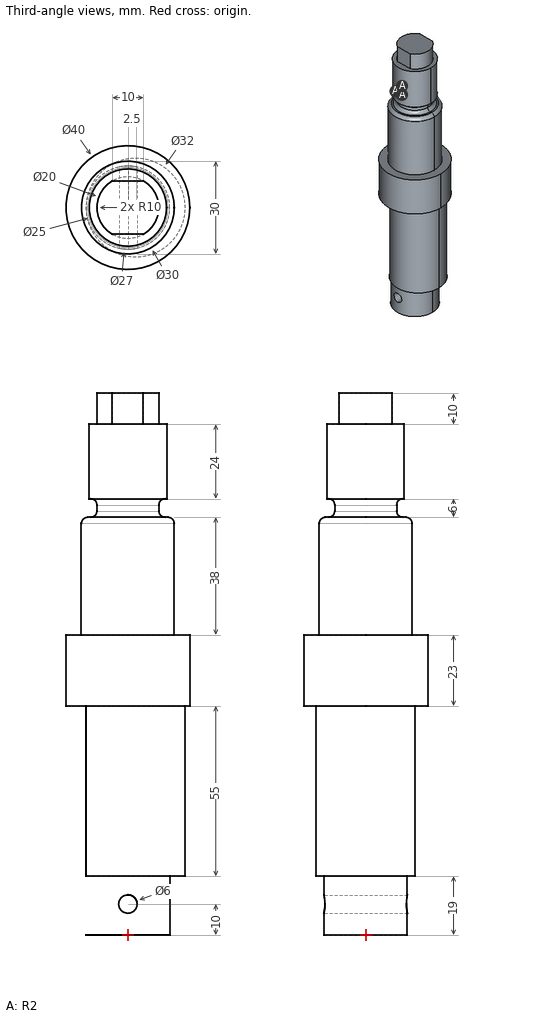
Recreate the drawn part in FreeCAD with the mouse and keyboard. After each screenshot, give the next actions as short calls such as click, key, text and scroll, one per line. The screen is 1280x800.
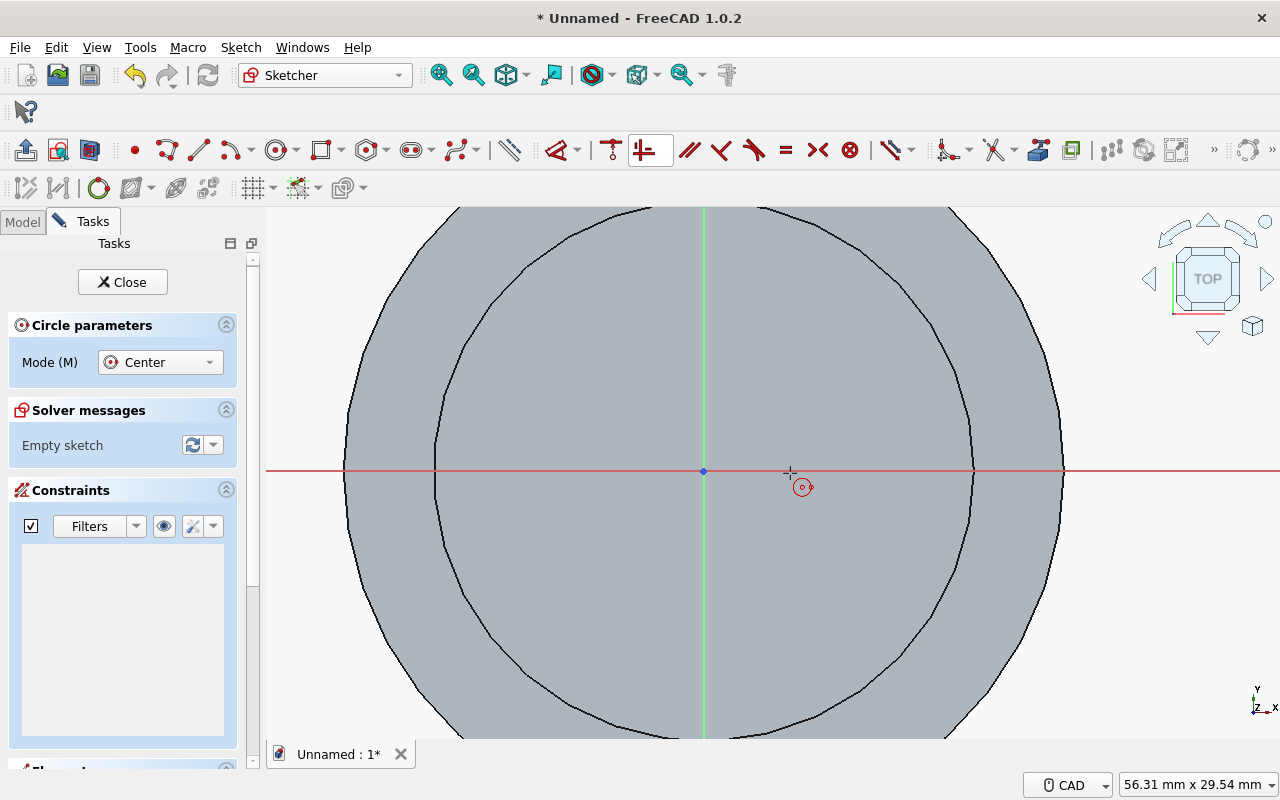
click(704, 471)
click(831, 344)
key(Escape)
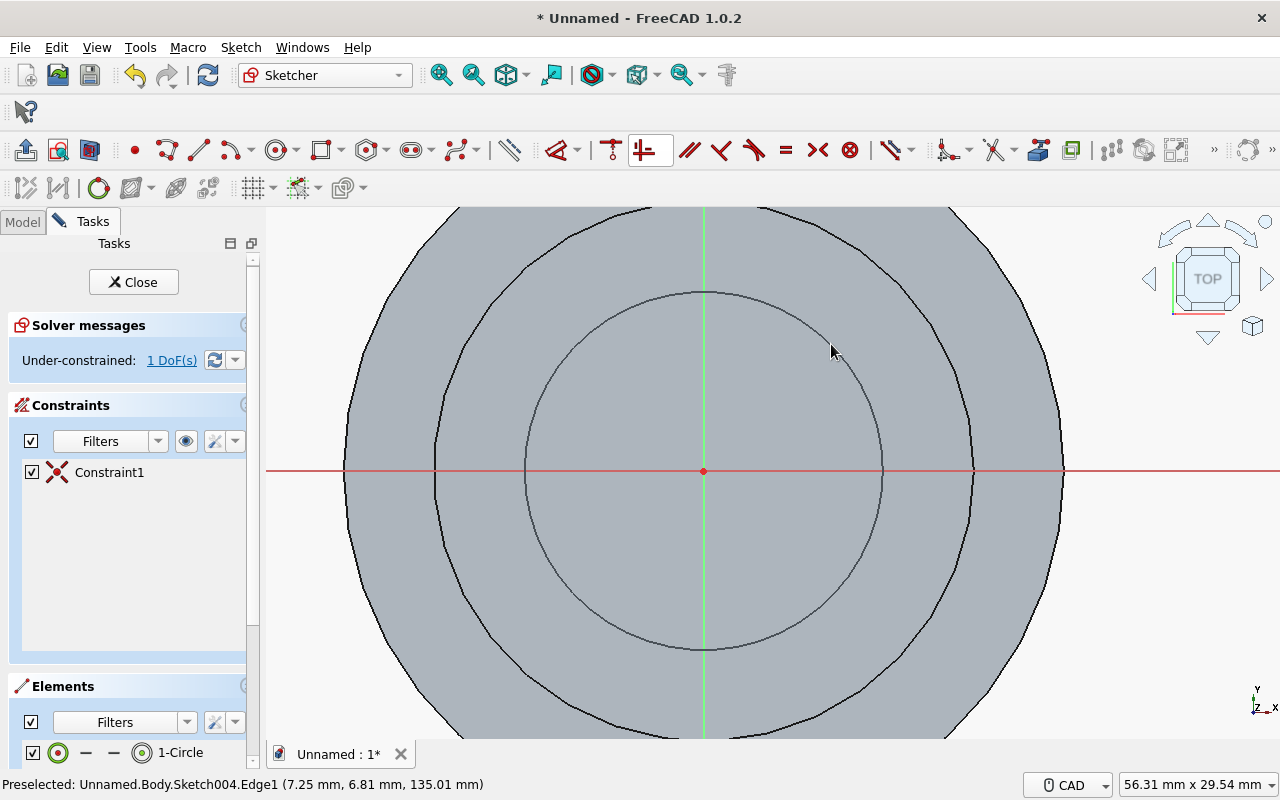
key(d)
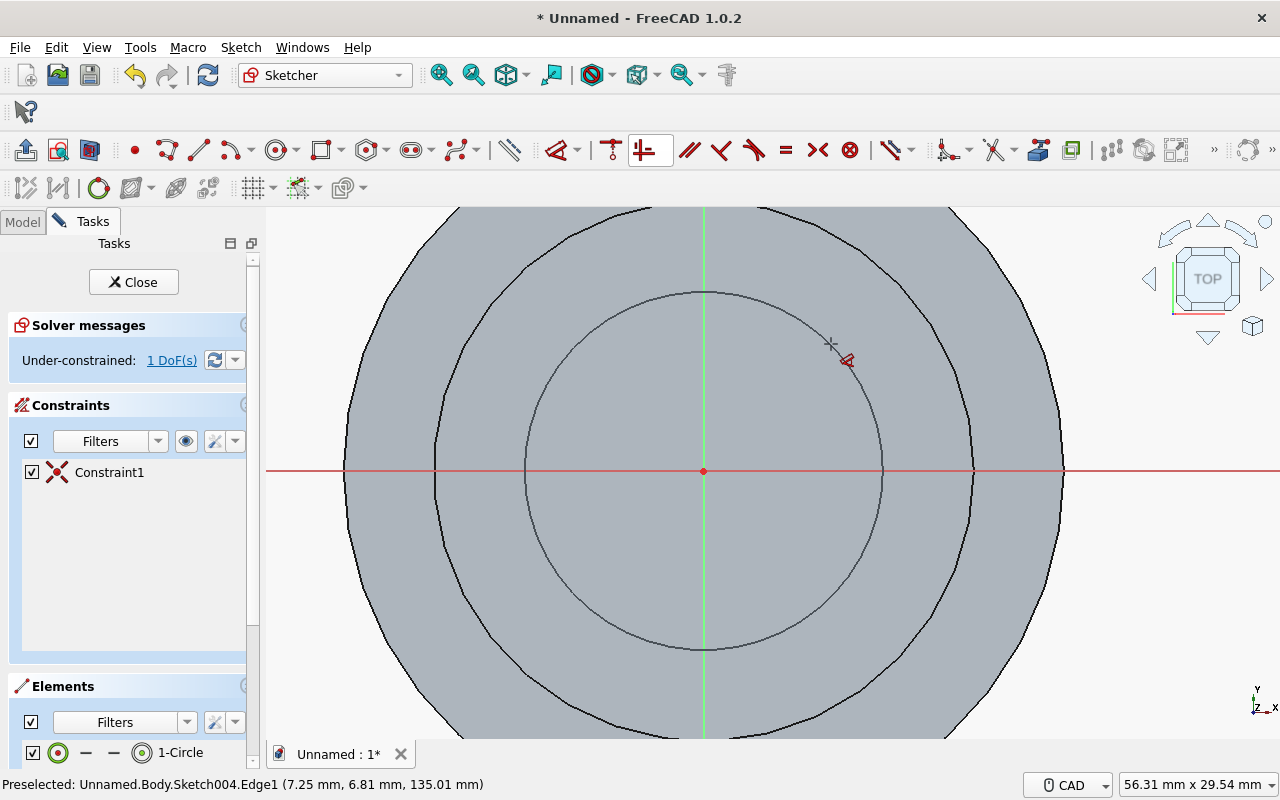
click(830, 344)
click(853, 321)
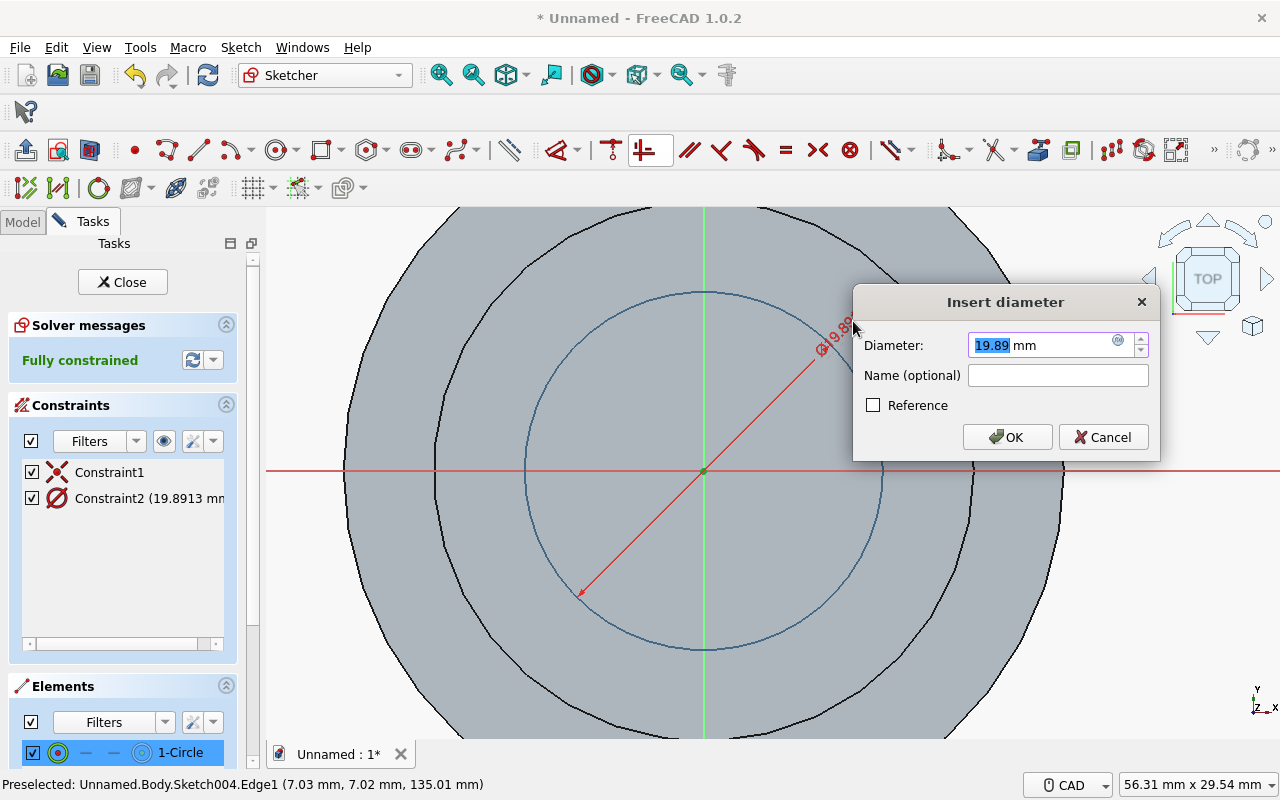
text(20)
key(Return)
key(Escape)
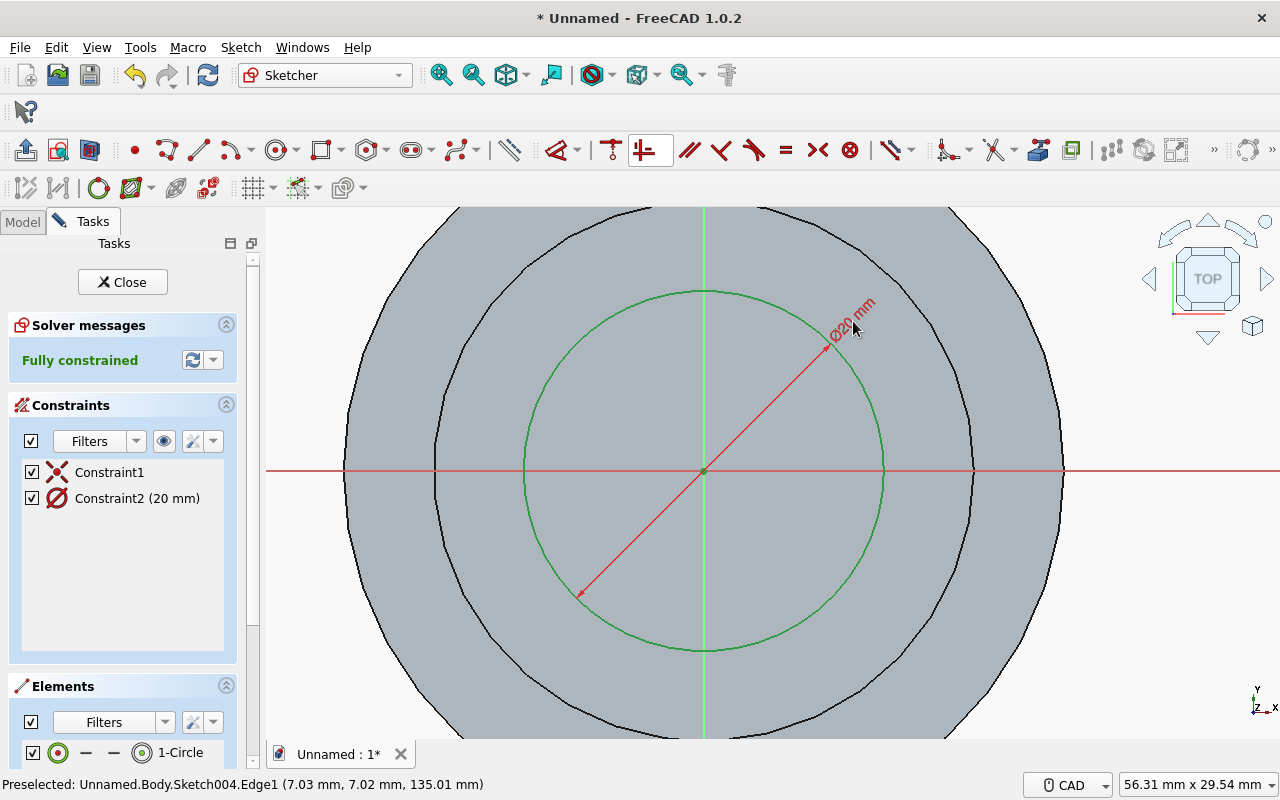
click(123, 282)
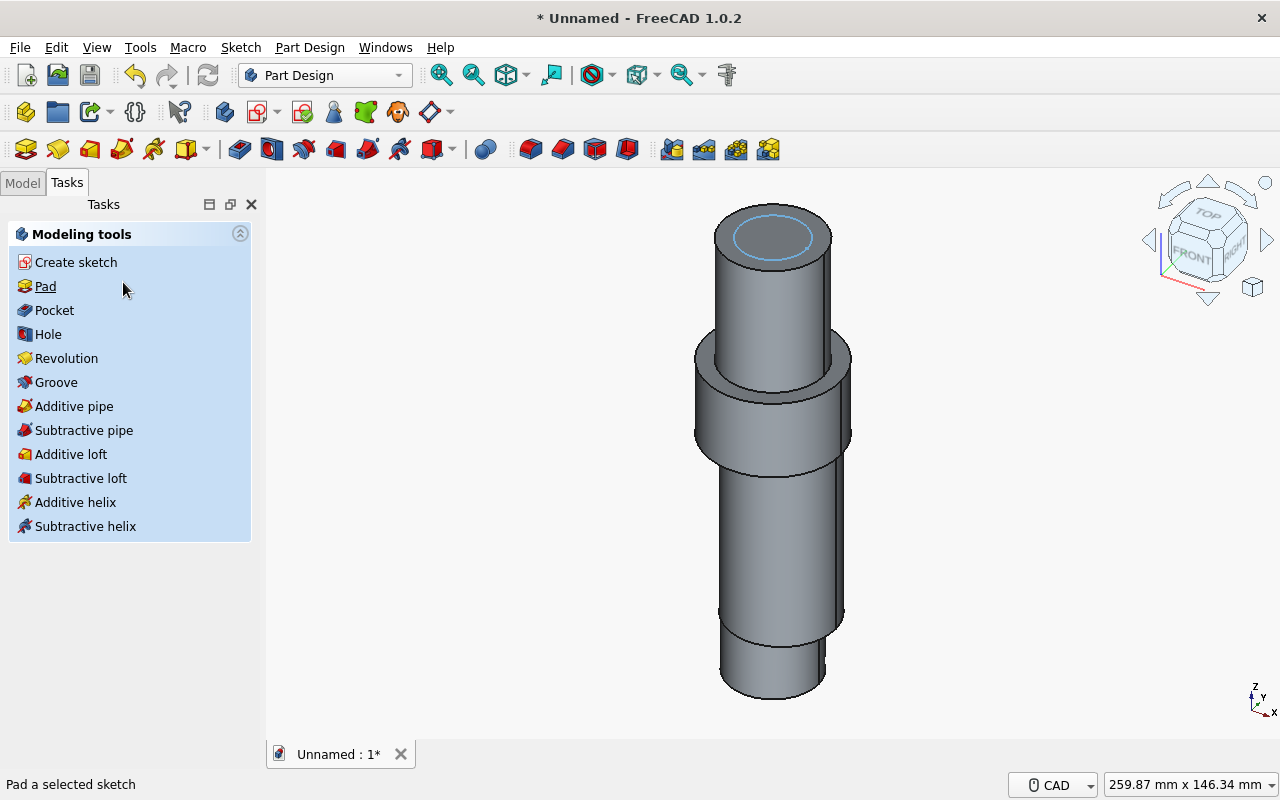
click(26, 150)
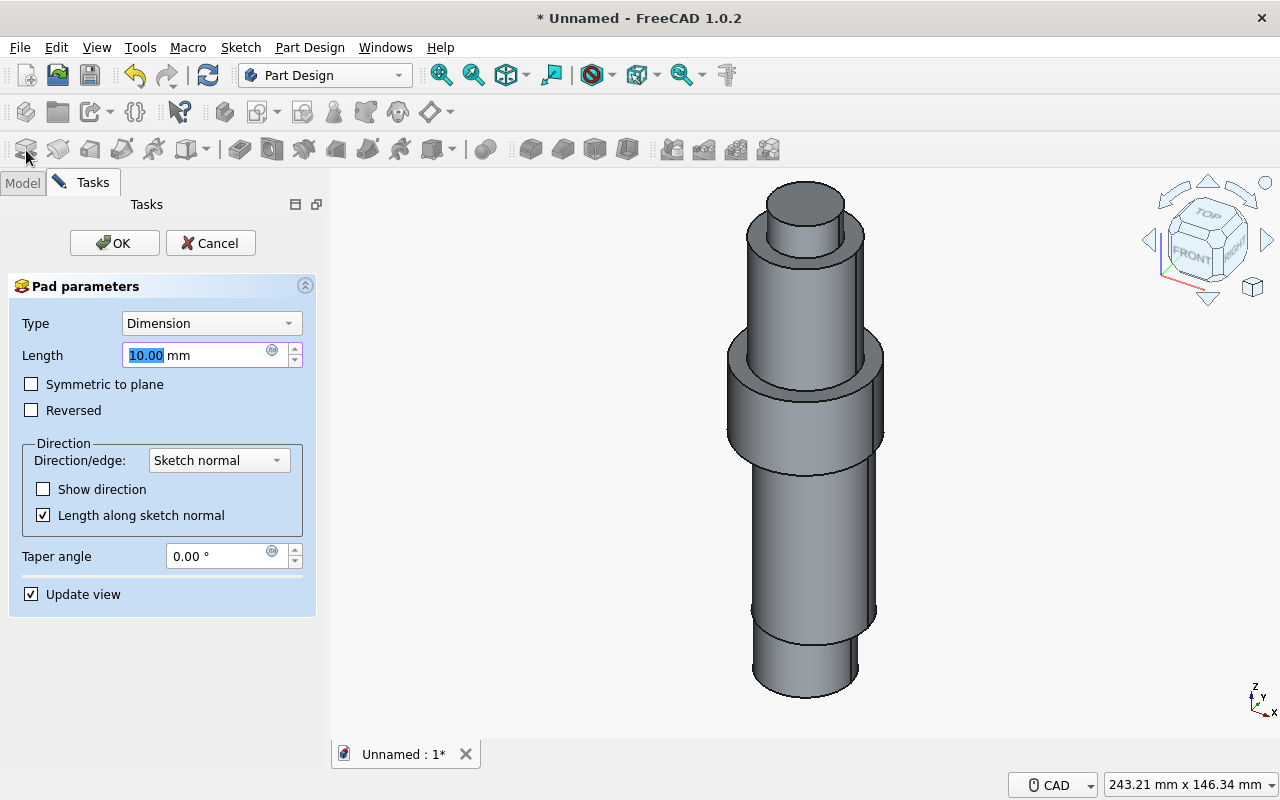
text(6)
key(Tab)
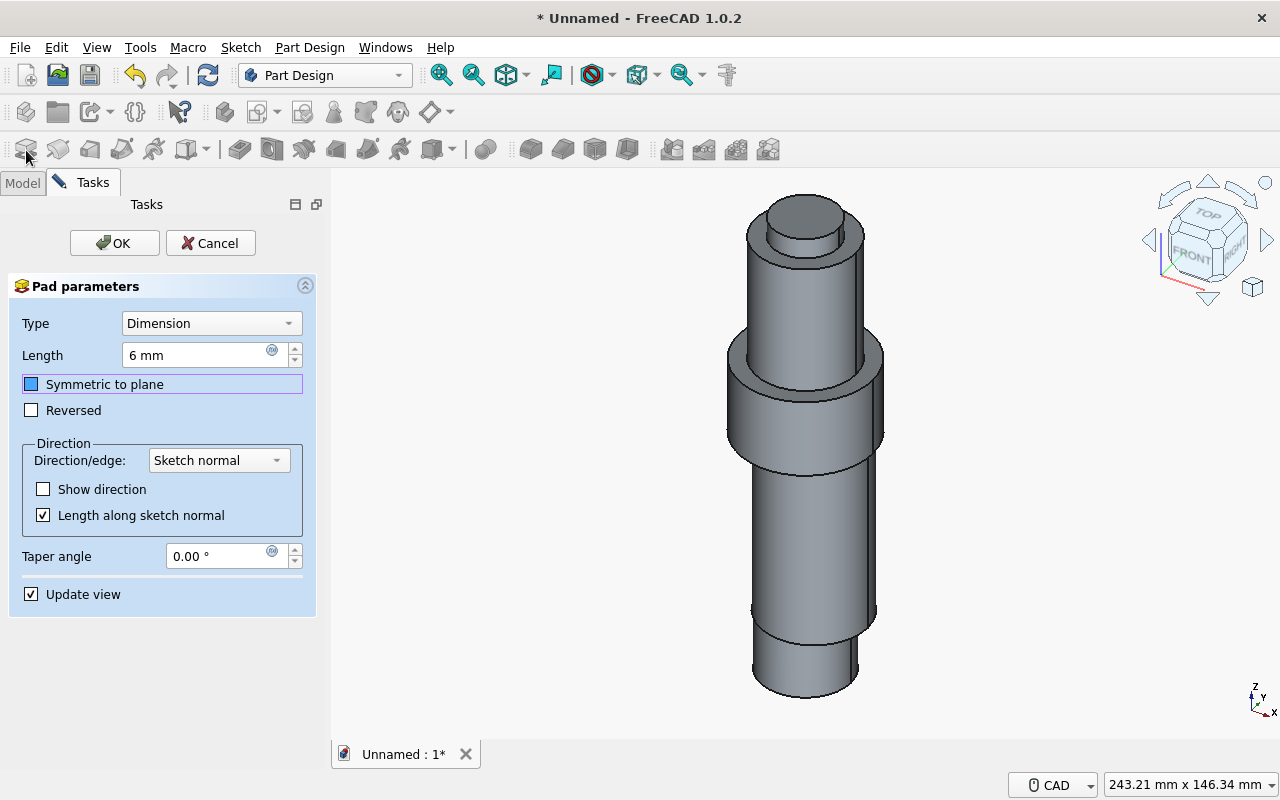
click(115, 243)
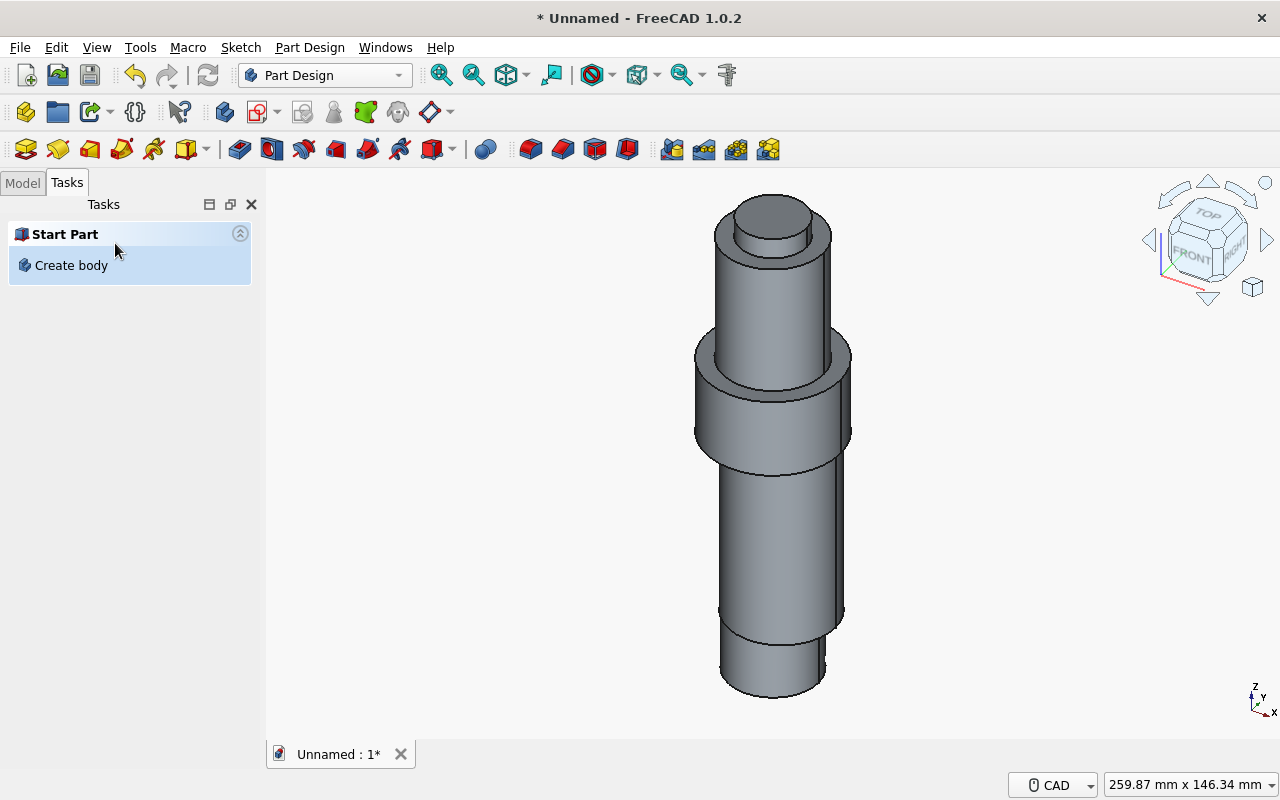
key(v)
key(f)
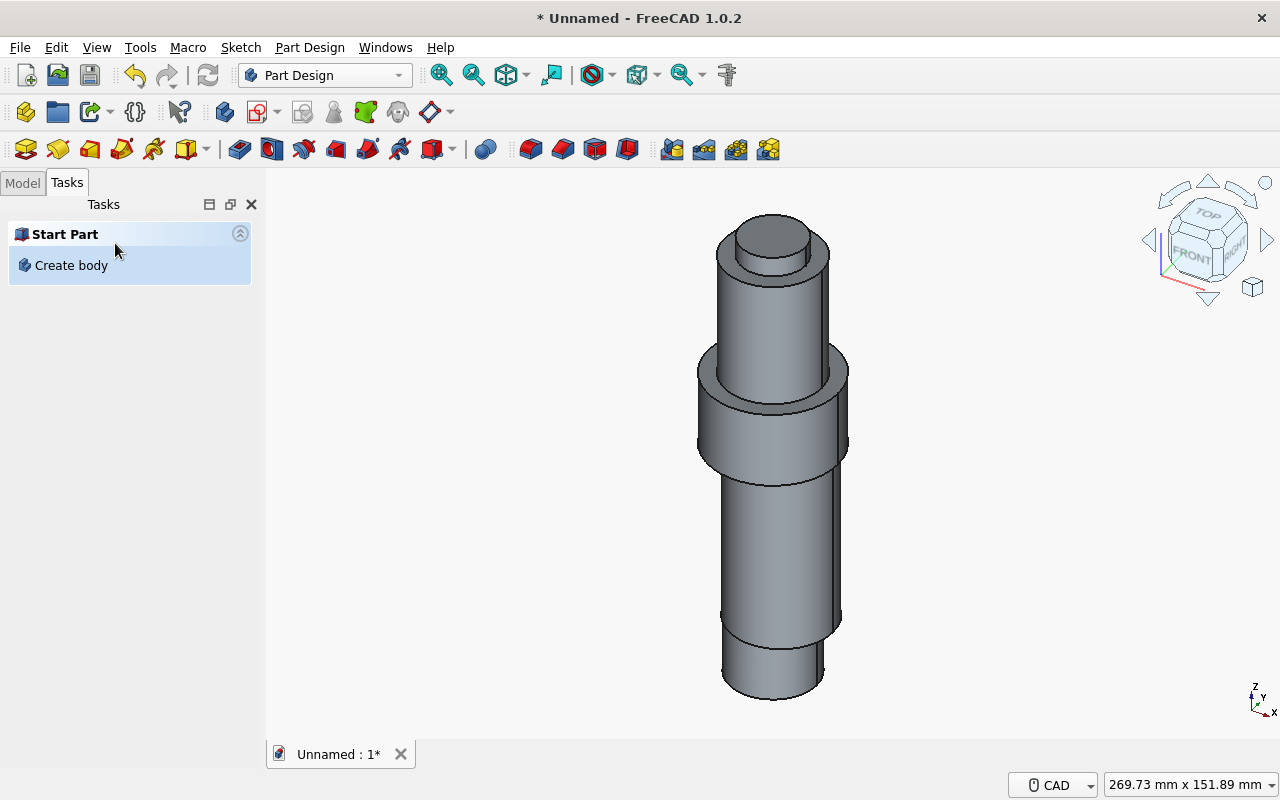
click(773, 235)